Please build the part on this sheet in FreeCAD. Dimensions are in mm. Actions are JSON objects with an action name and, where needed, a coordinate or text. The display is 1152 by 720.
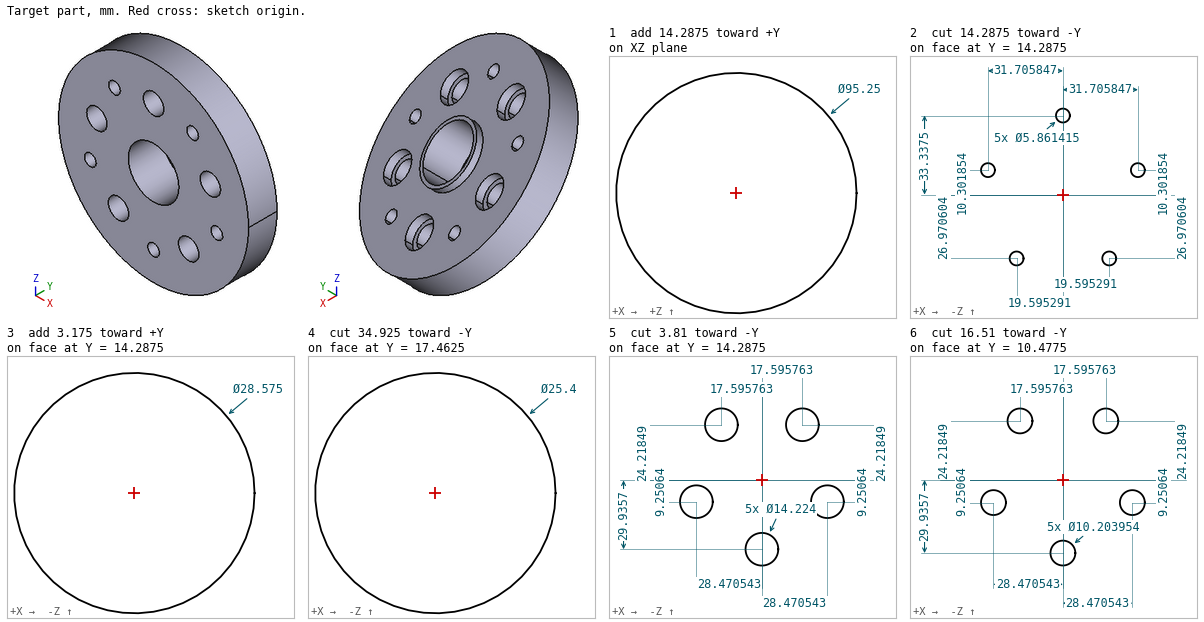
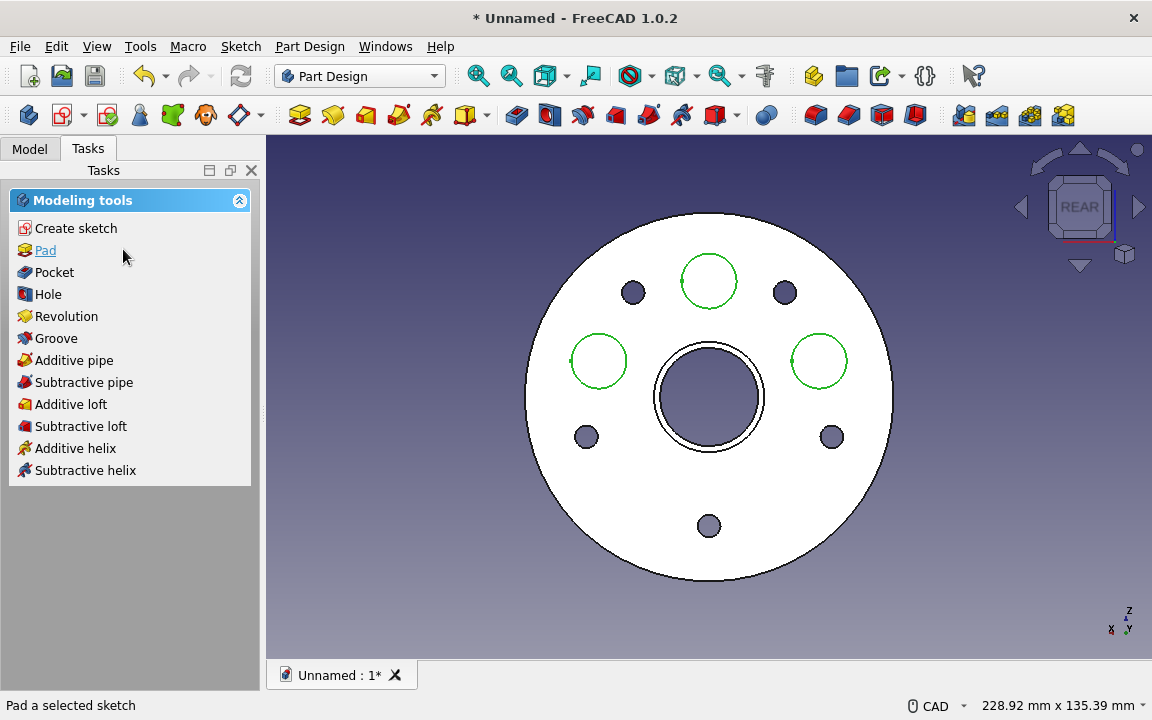
{"action": "left_click", "coordinate": [517, 116]}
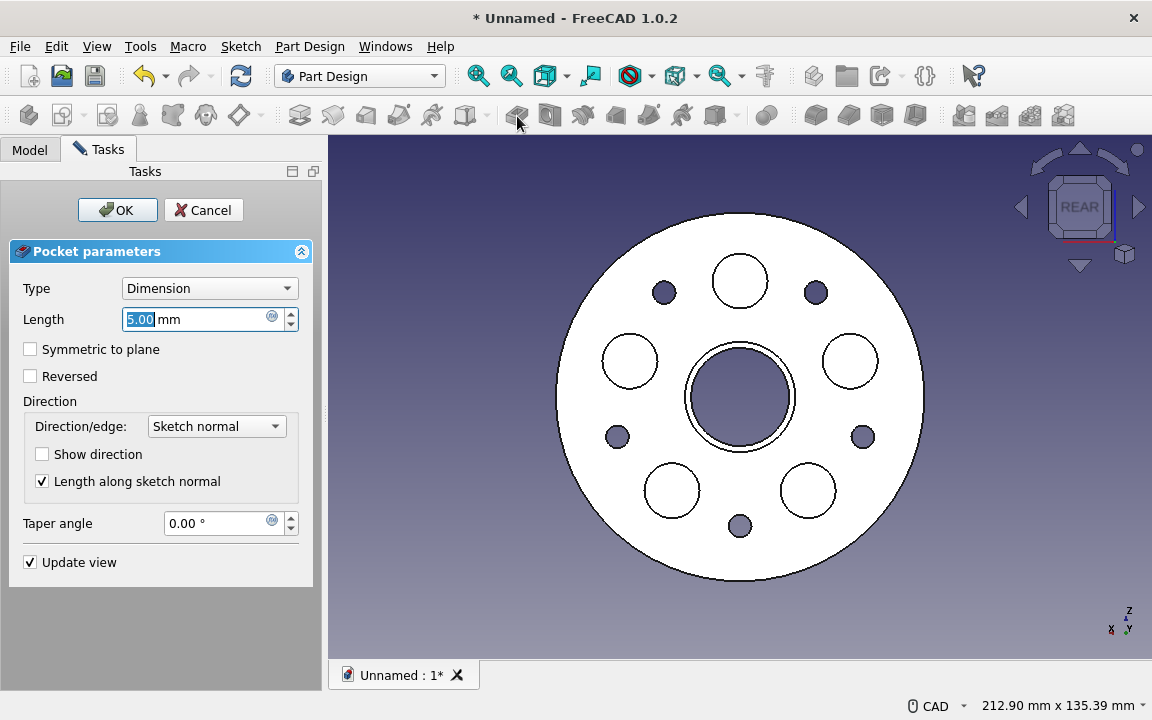
{"action": "type", "text": "3.81"}
{"action": "key", "text": "Tab"}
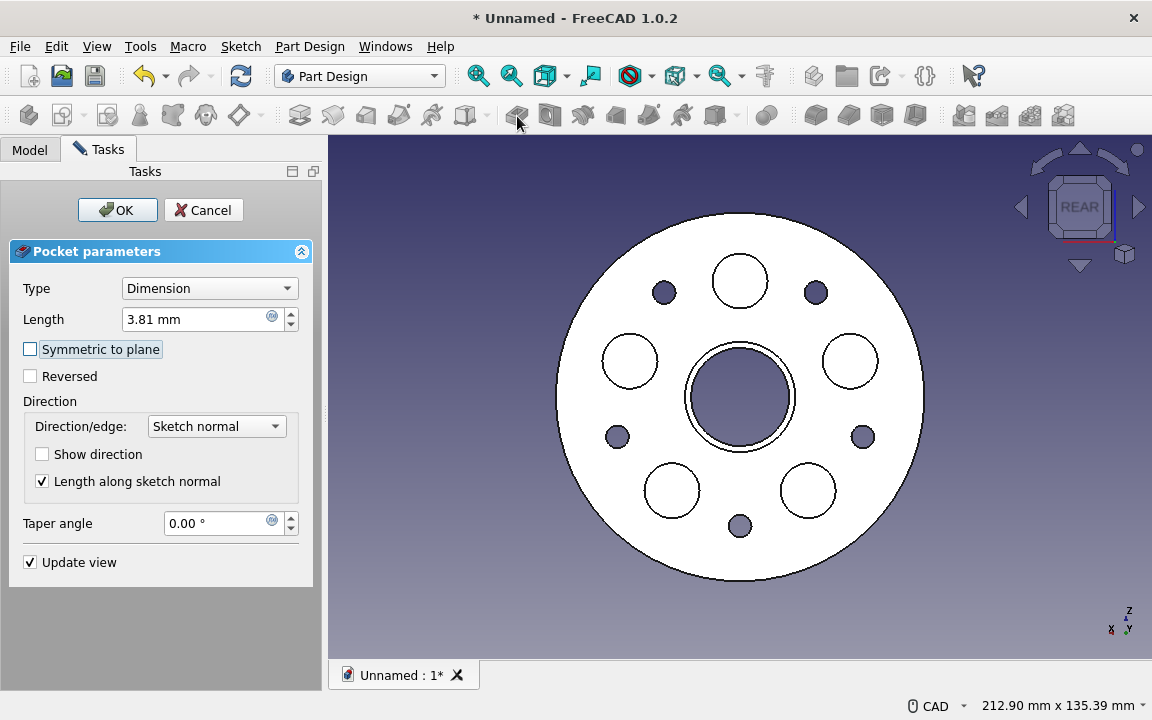
{"action": "left_click", "coordinate": [118, 210]}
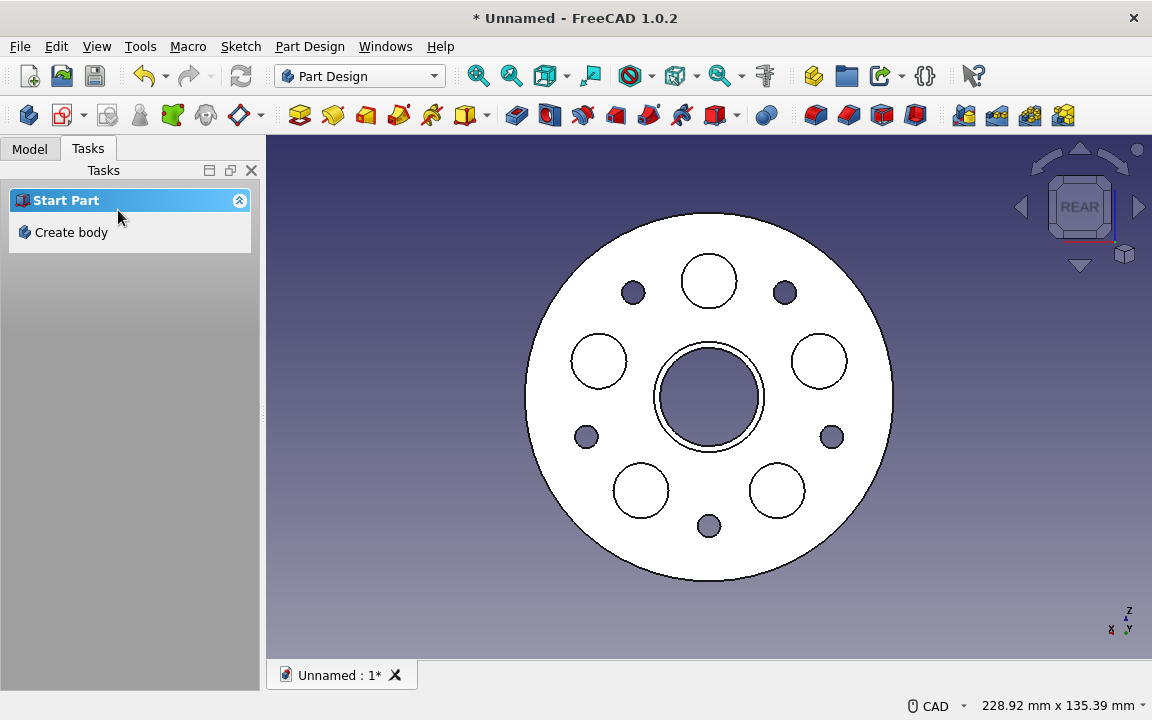
{"action": "left_click", "coordinate": [599, 360]}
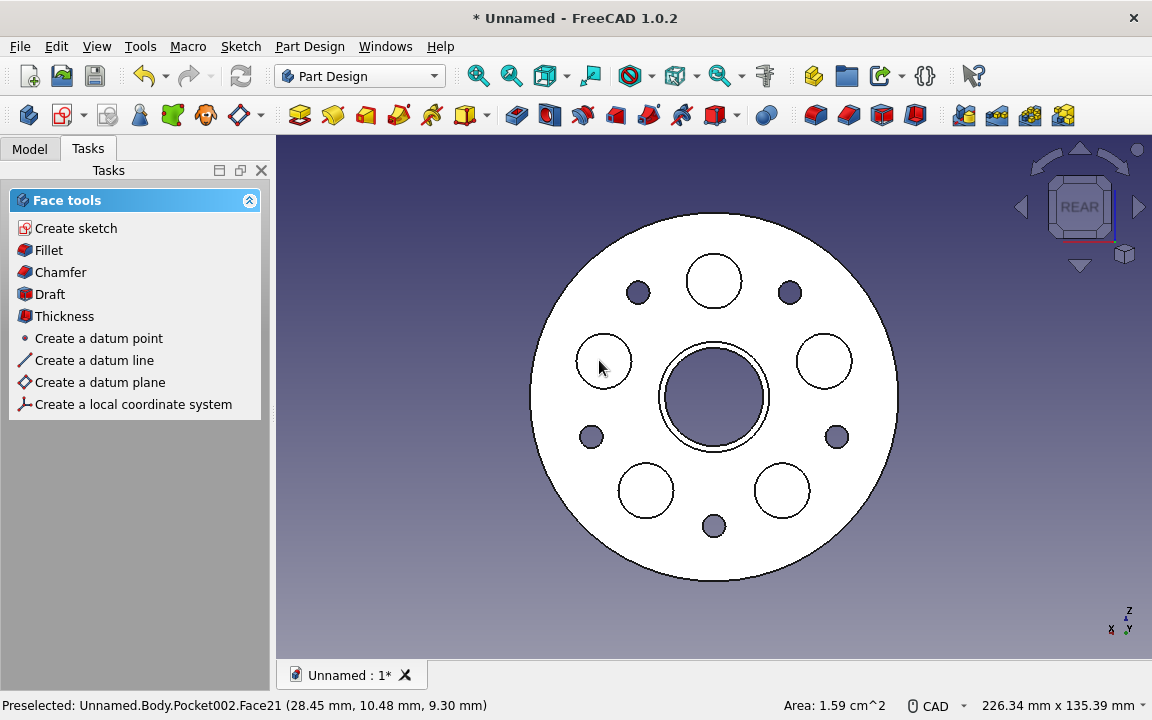
{"action": "left_click", "coordinate": [62, 116]}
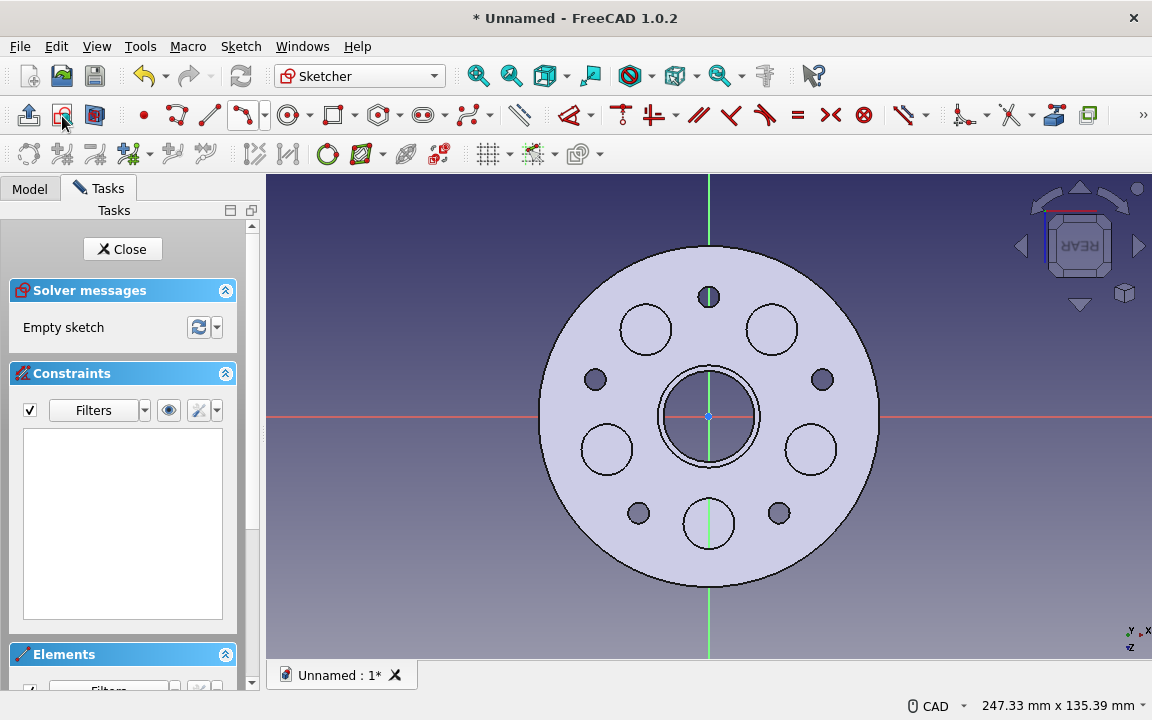
{"action": "left_click", "coordinate": [288, 116]}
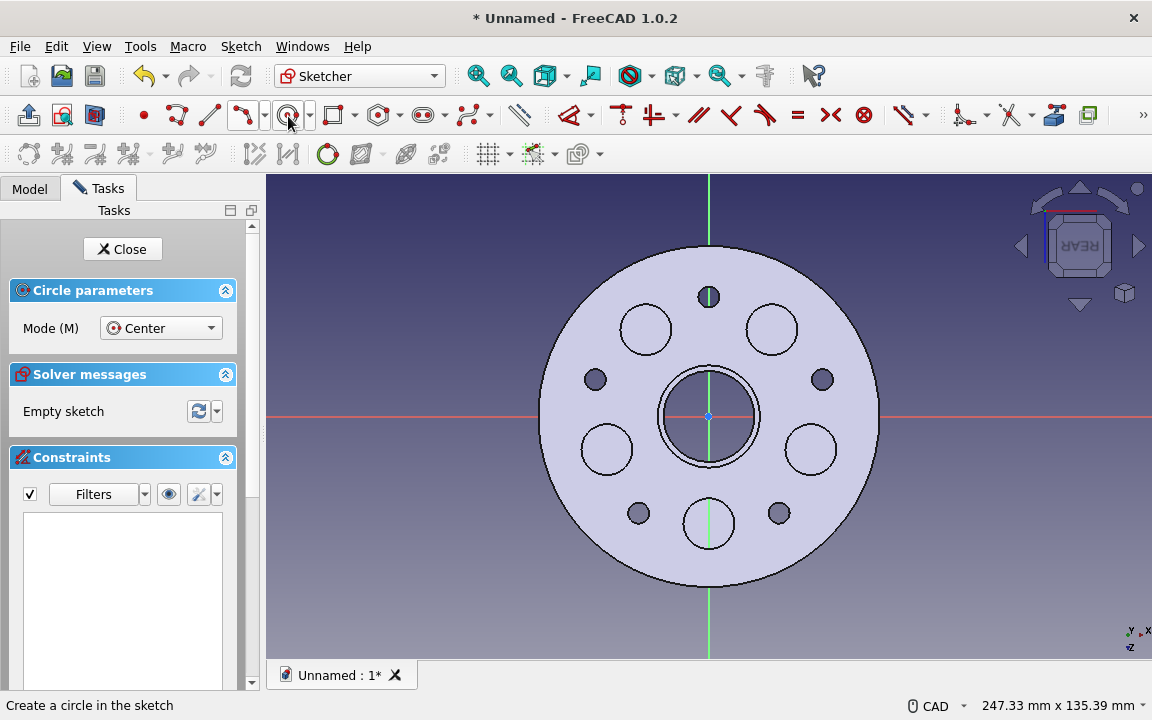
{"action": "scroll", "coordinate": [709, 524], "scroll_direction": "up", "scroll_amount": 2}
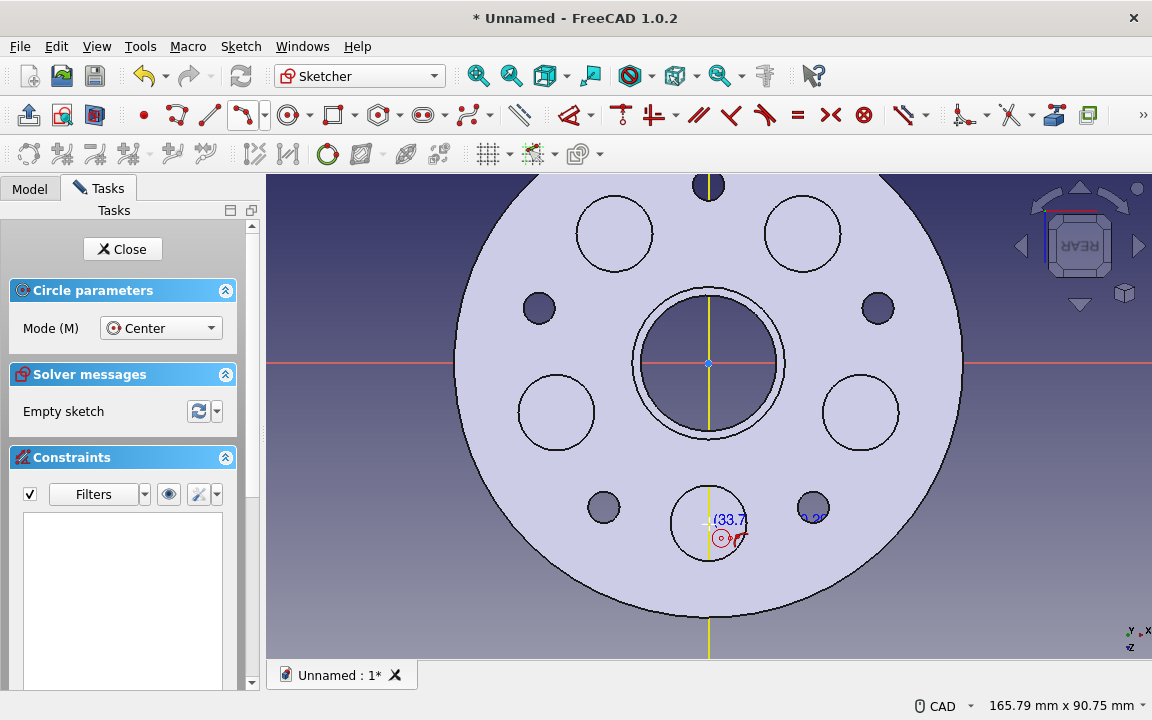
{"action": "left_click", "coordinate": [709, 523]}
{"action": "mouse_move", "coordinate": [728, 504]}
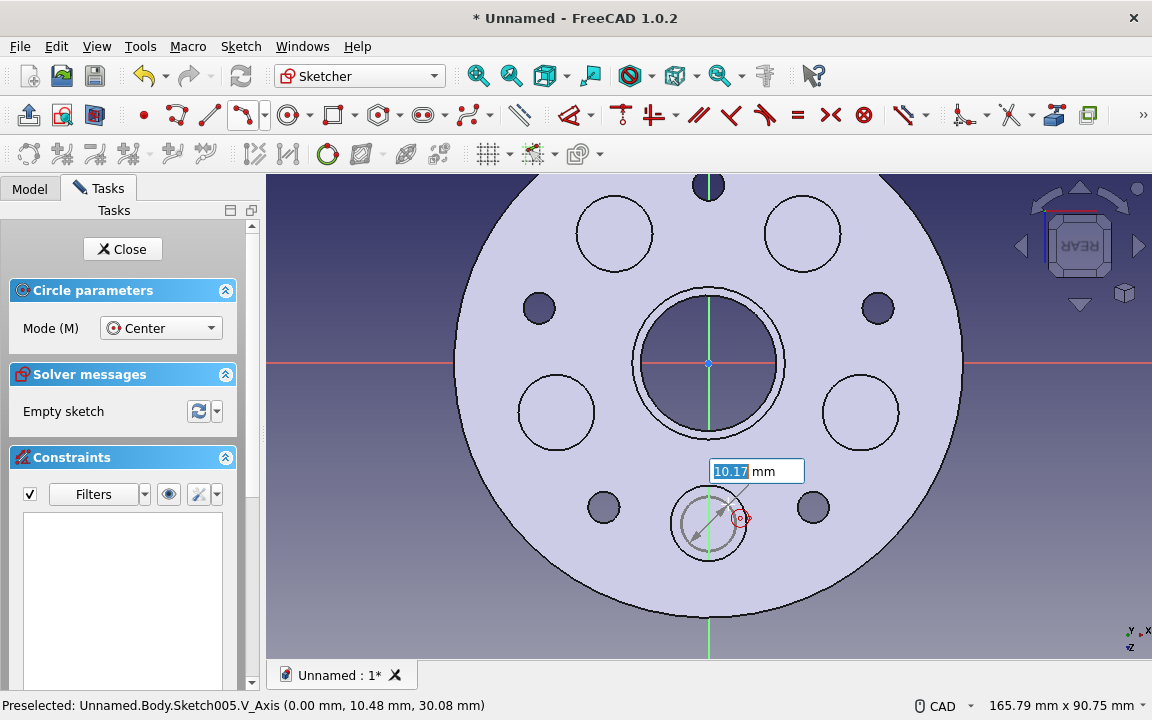
{"action": "type", "text": "10.203954"}
{"action": "key", "text": "Return"}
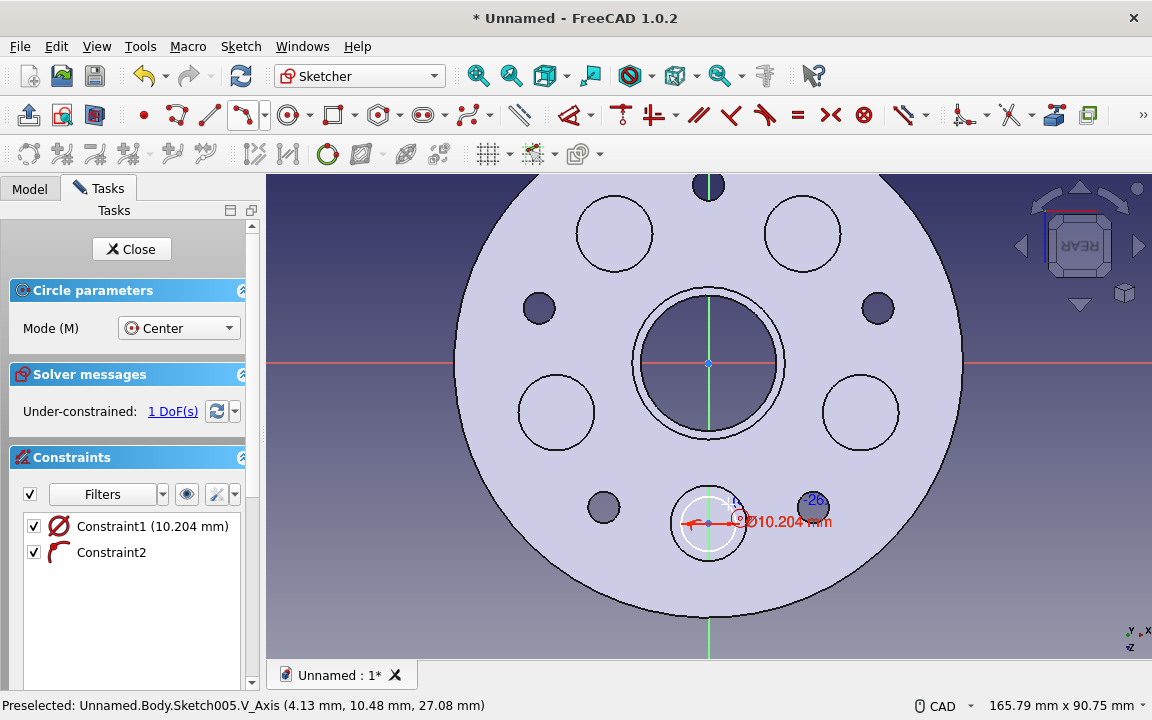
{"action": "left_click", "coordinate": [556, 413]}
{"action": "mouse_move", "coordinate": [576, 393]}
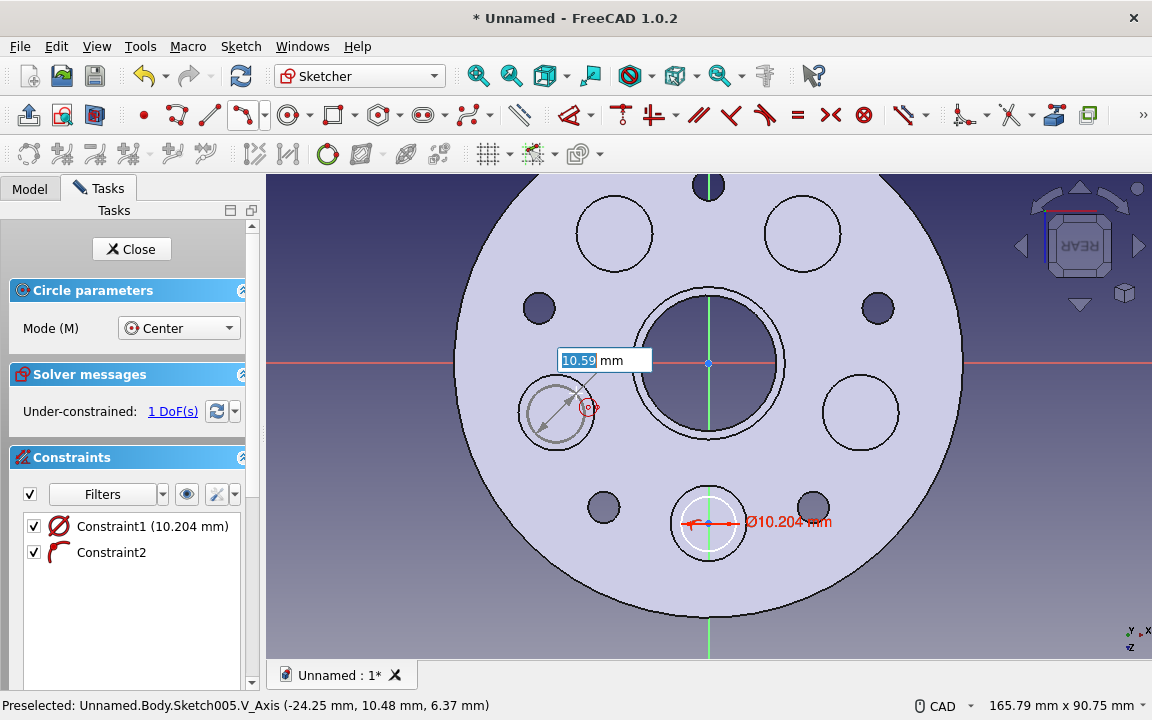
{"action": "type", "text": "10.203954"}
{"action": "key", "text": "Return"}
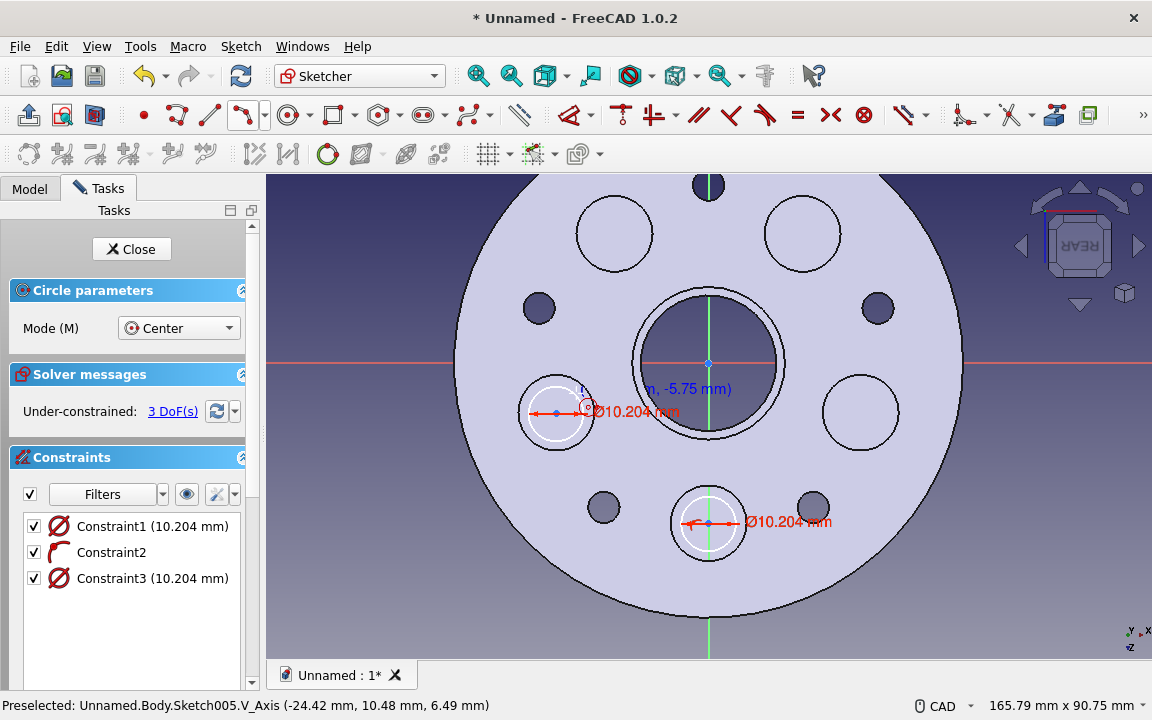
{"action": "left_click", "coordinate": [615, 234]}
{"action": "mouse_move", "coordinate": [634, 215]}